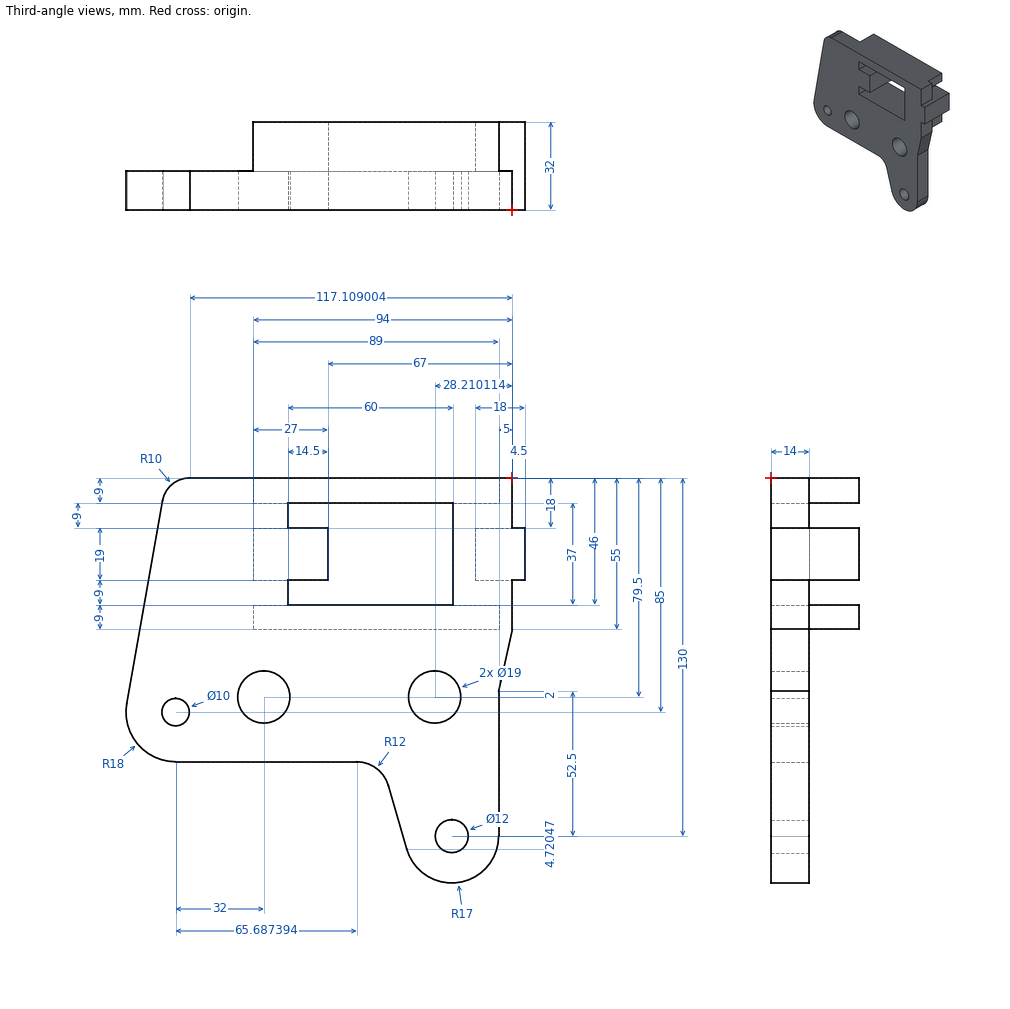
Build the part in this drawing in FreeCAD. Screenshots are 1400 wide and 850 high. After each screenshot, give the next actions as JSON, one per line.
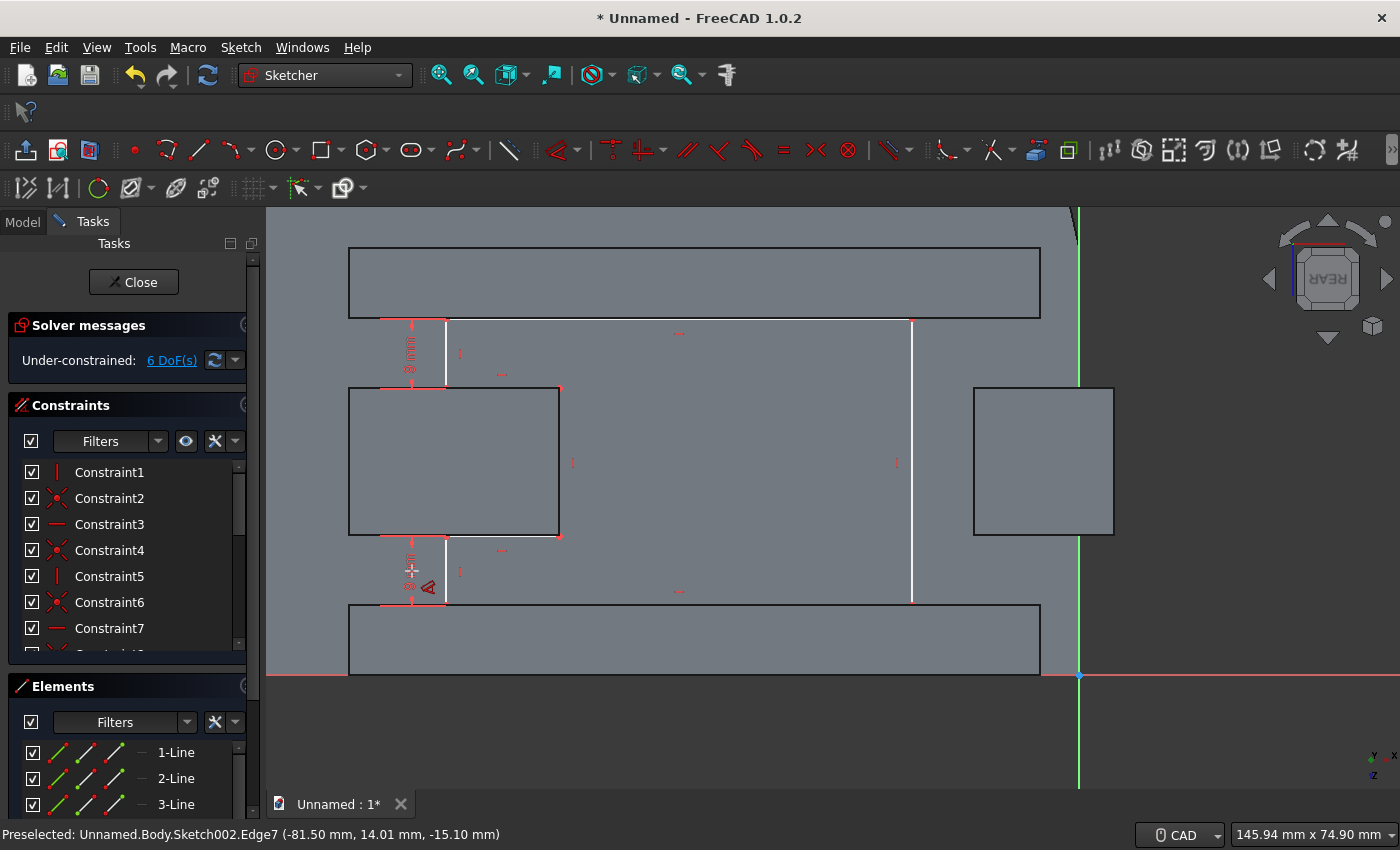
{"action": "left_click", "coordinate": [912, 520]}
{"action": "left_click", "coordinate": [946, 462]}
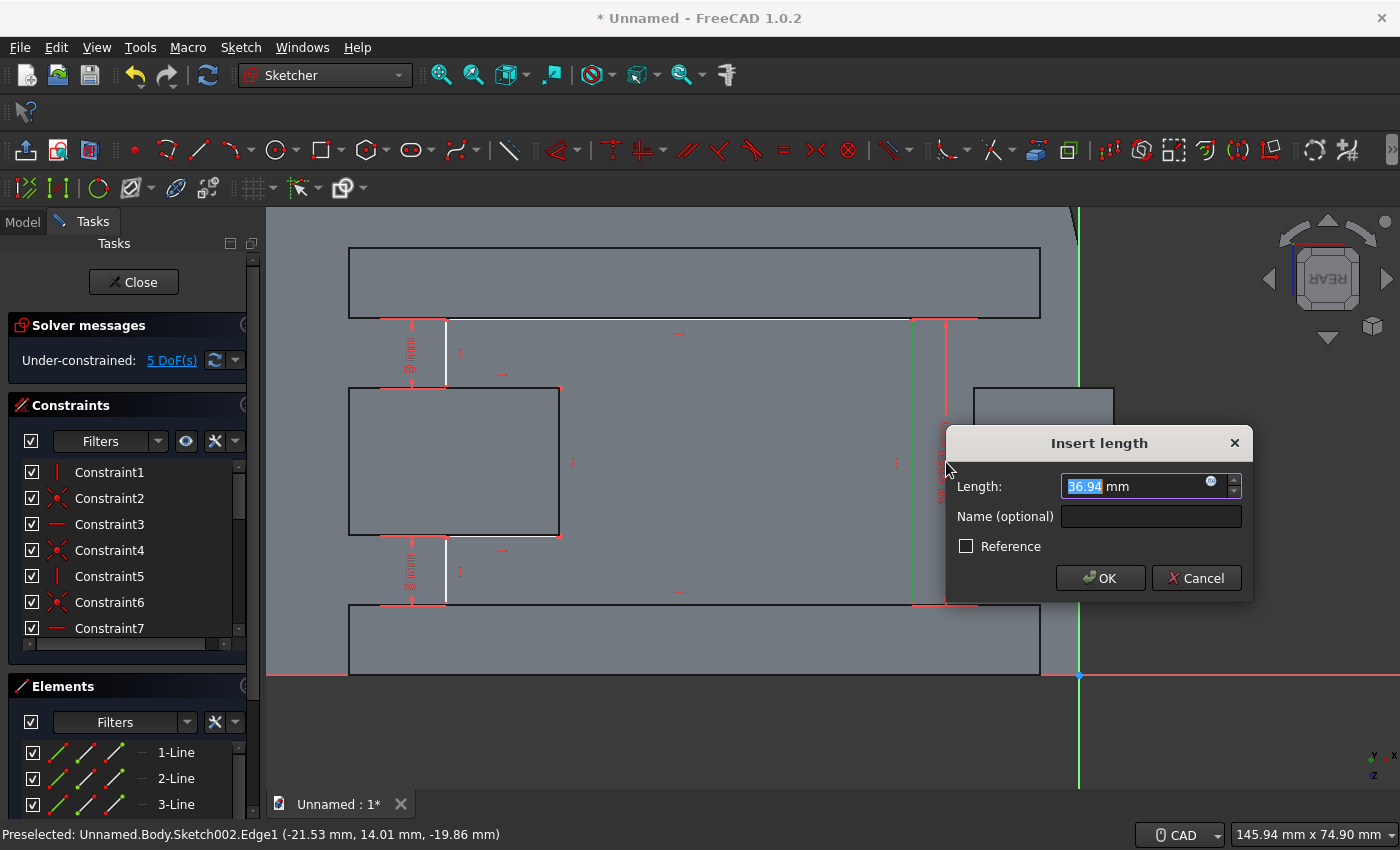
{"action": "type", "text": "37"}
{"action": "key", "text": "Return"}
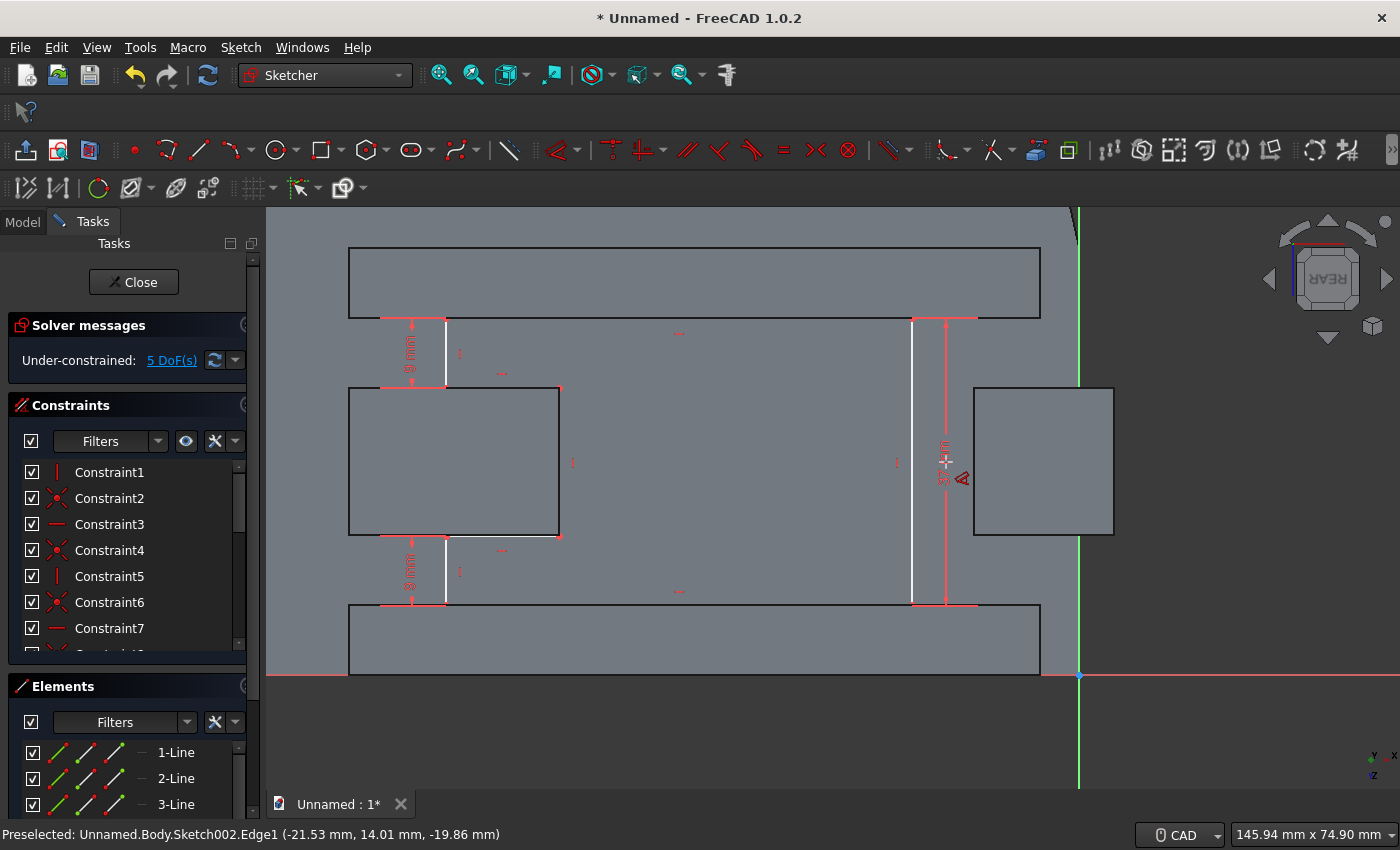
{"action": "left_click", "coordinate": [772, 318]}
{"action": "left_click", "coordinate": [679, 284]}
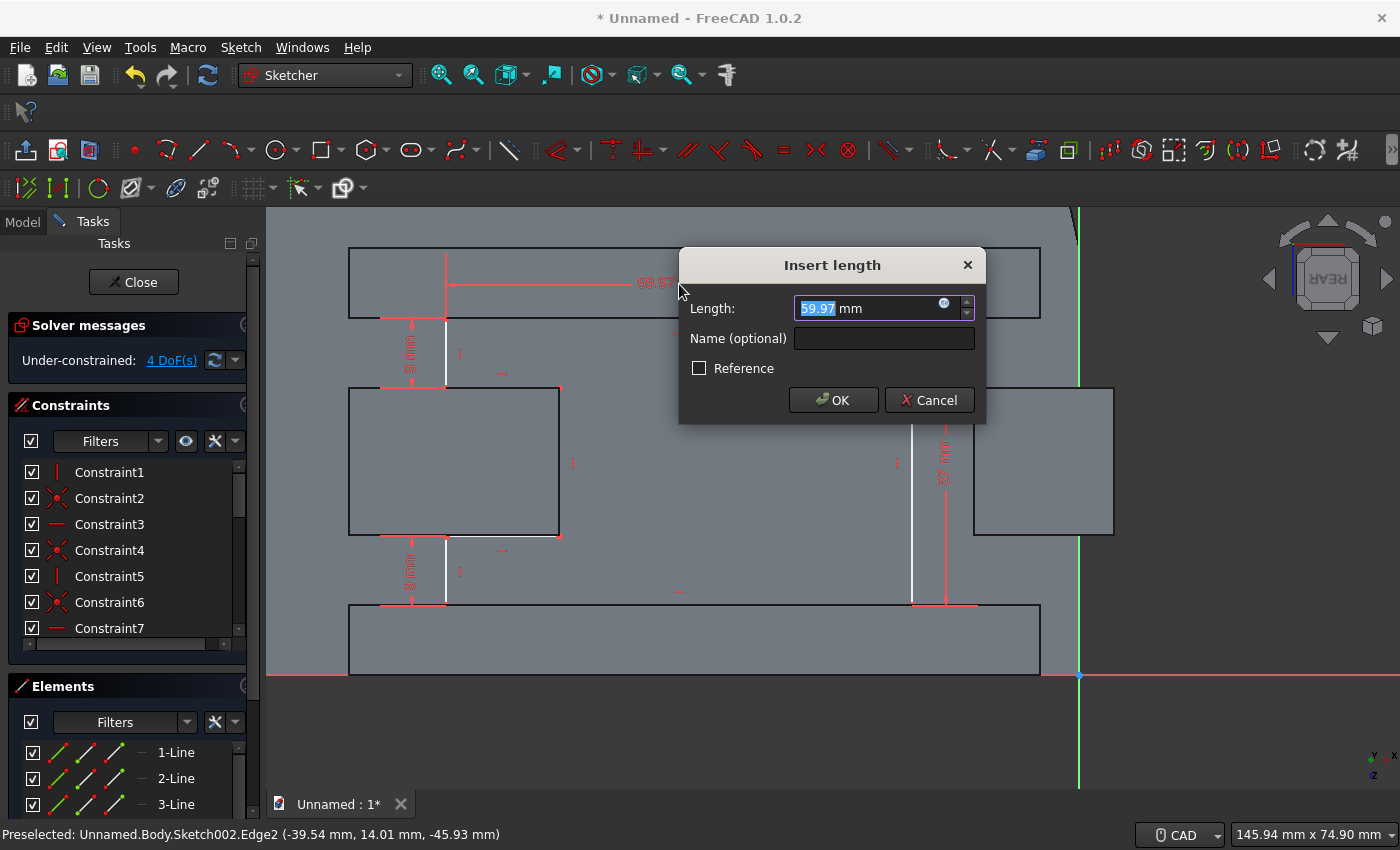
{"action": "type", "text": "60"}
{"action": "key", "text": "Return"}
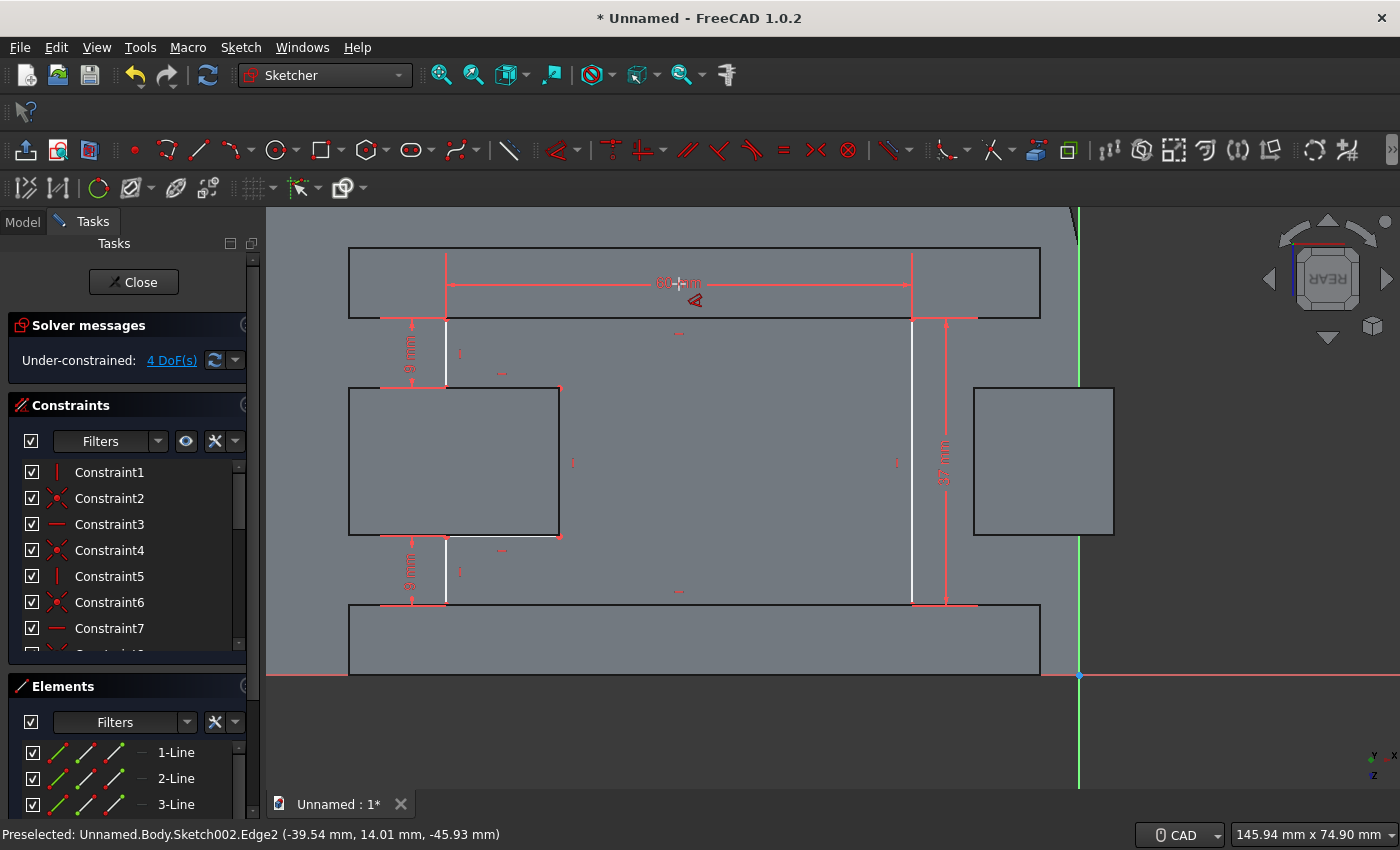
{"action": "left_click", "coordinate": [586, 606]}
{"action": "left_click", "coordinate": [679, 640]}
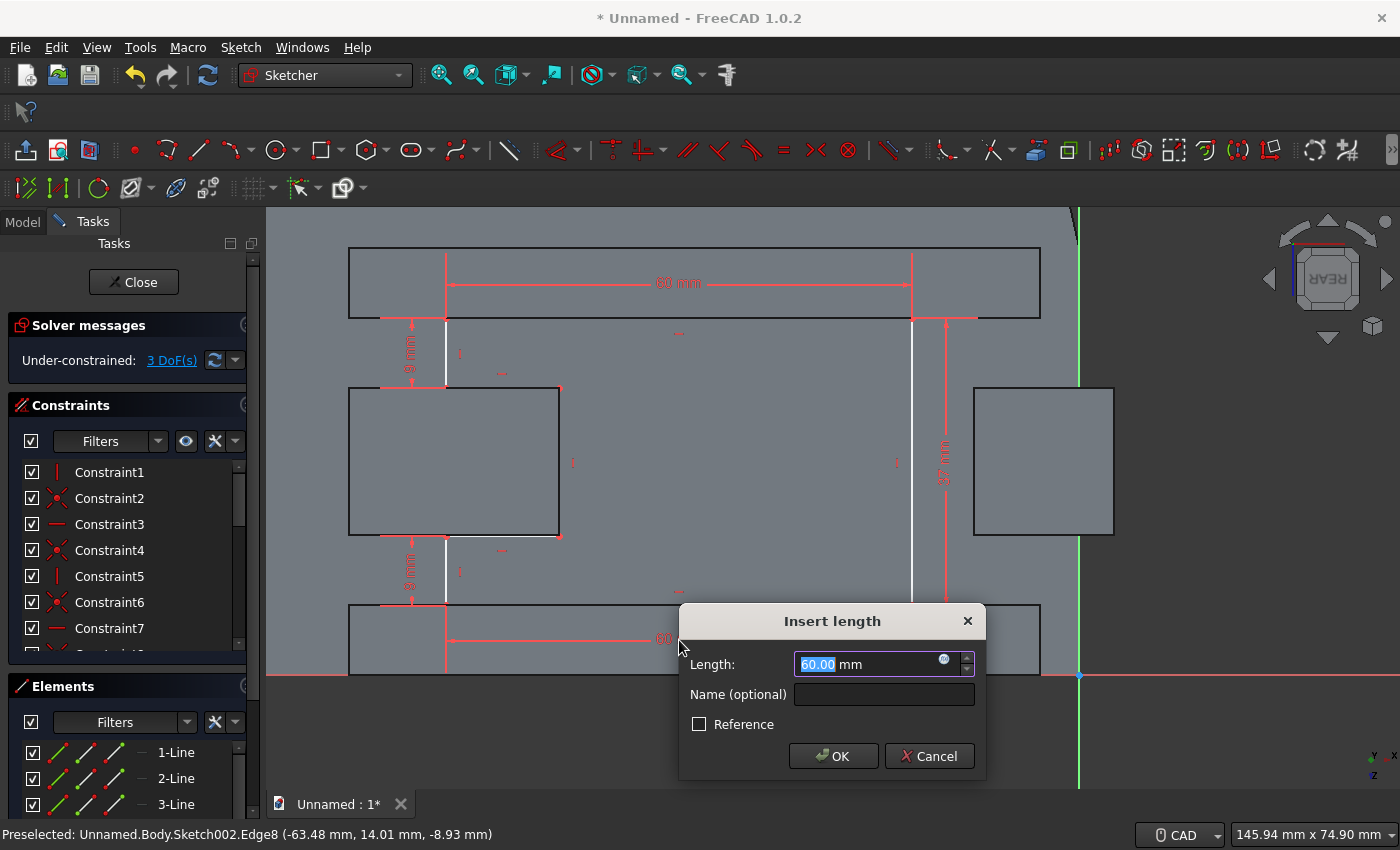
{"action": "type", "text": "60"}
{"action": "key", "text": "Return"}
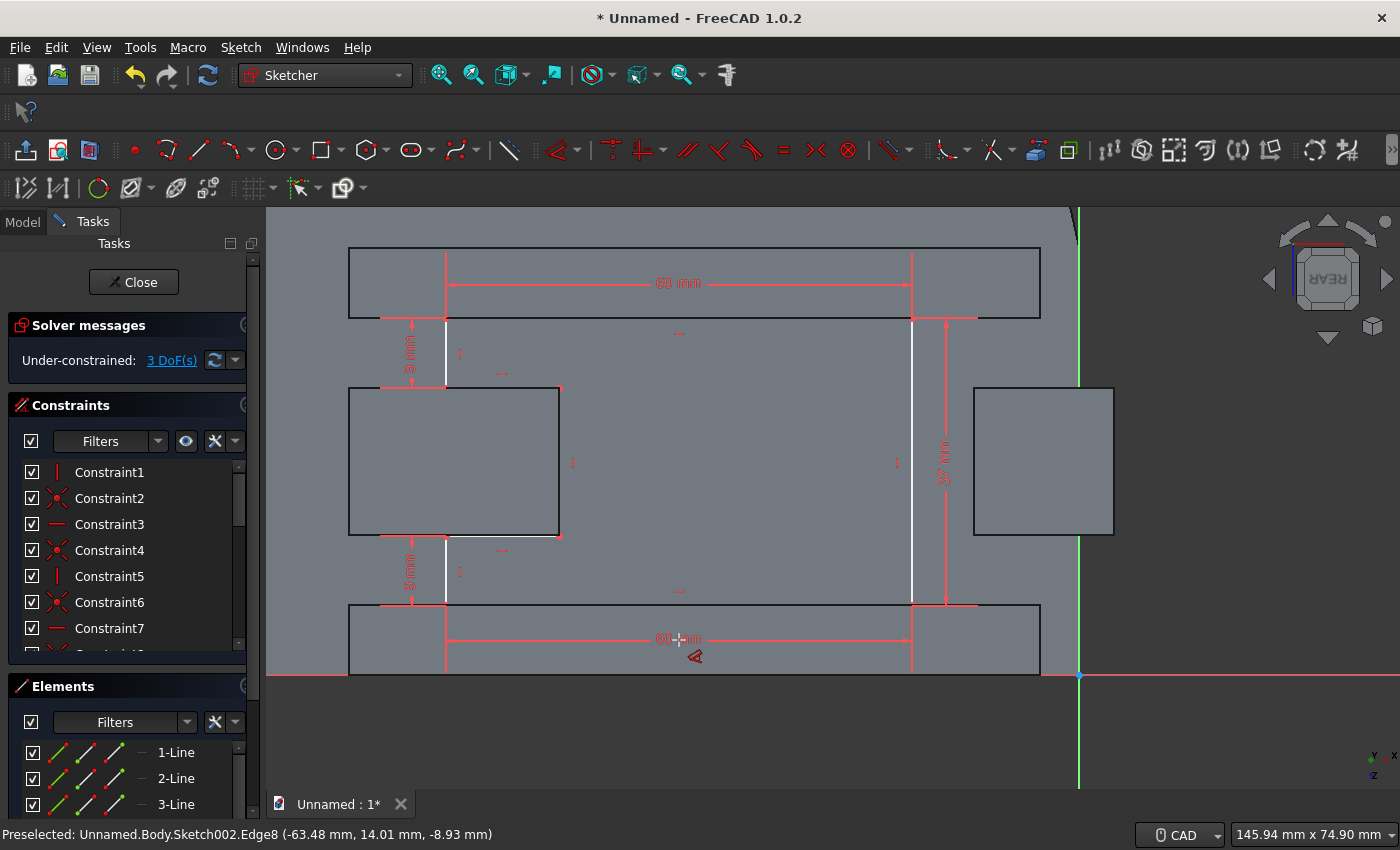
{"action": "left_click", "coordinate": [912, 606]}
{"action": "left_click", "coordinate": [1113, 641]}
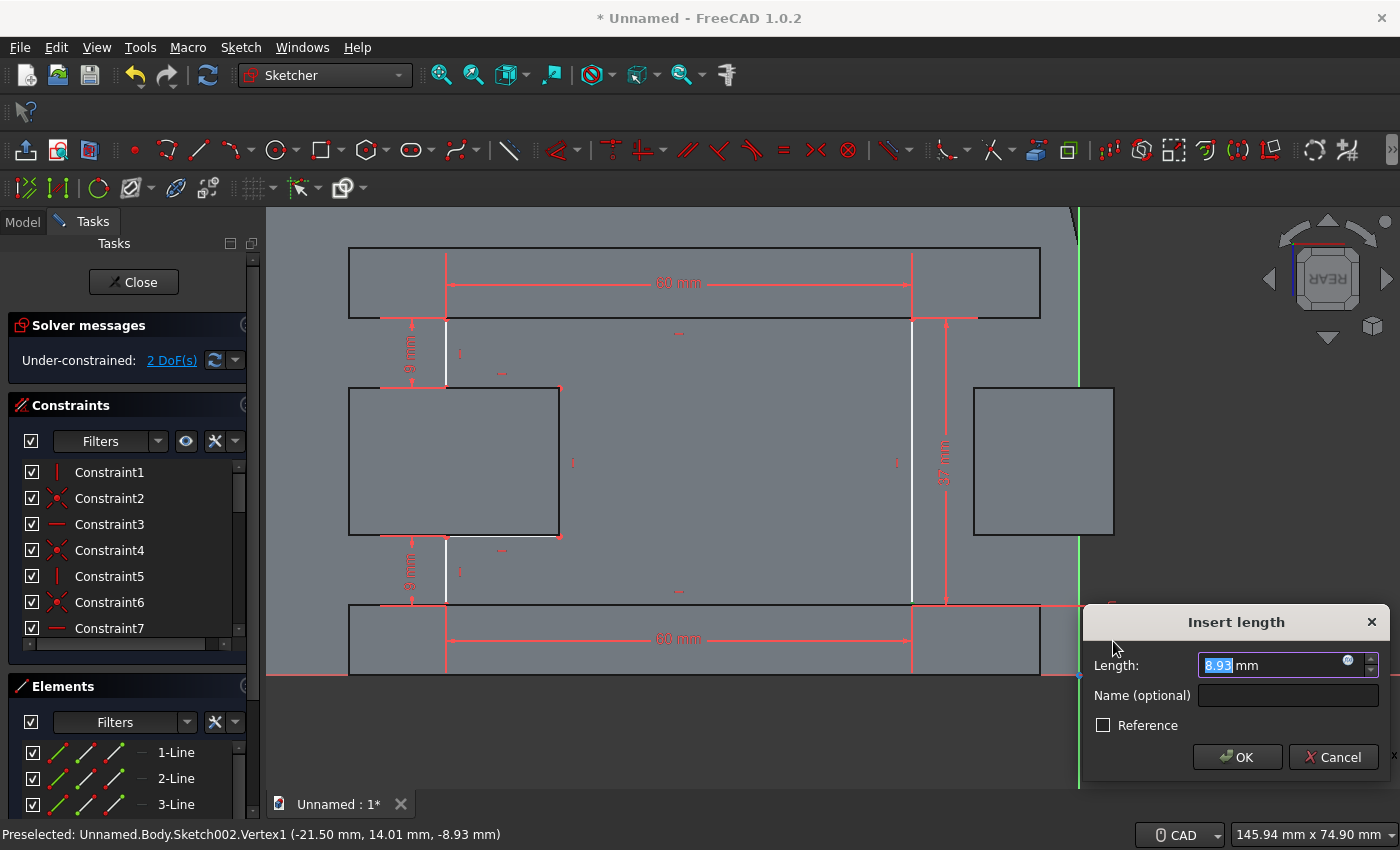
{"action": "type", "text": "9"}
{"action": "key", "text": "Return"}